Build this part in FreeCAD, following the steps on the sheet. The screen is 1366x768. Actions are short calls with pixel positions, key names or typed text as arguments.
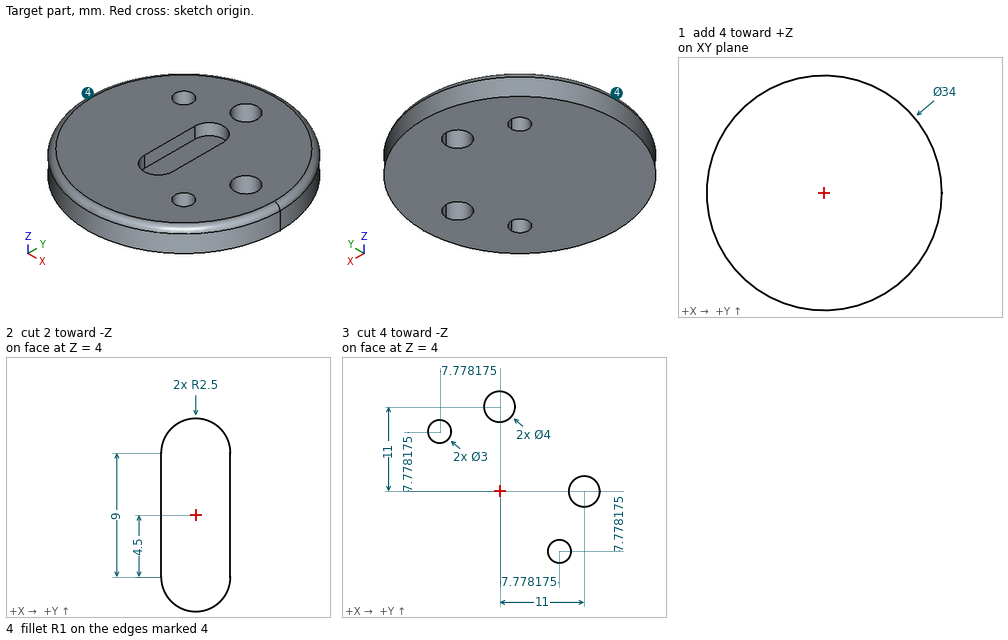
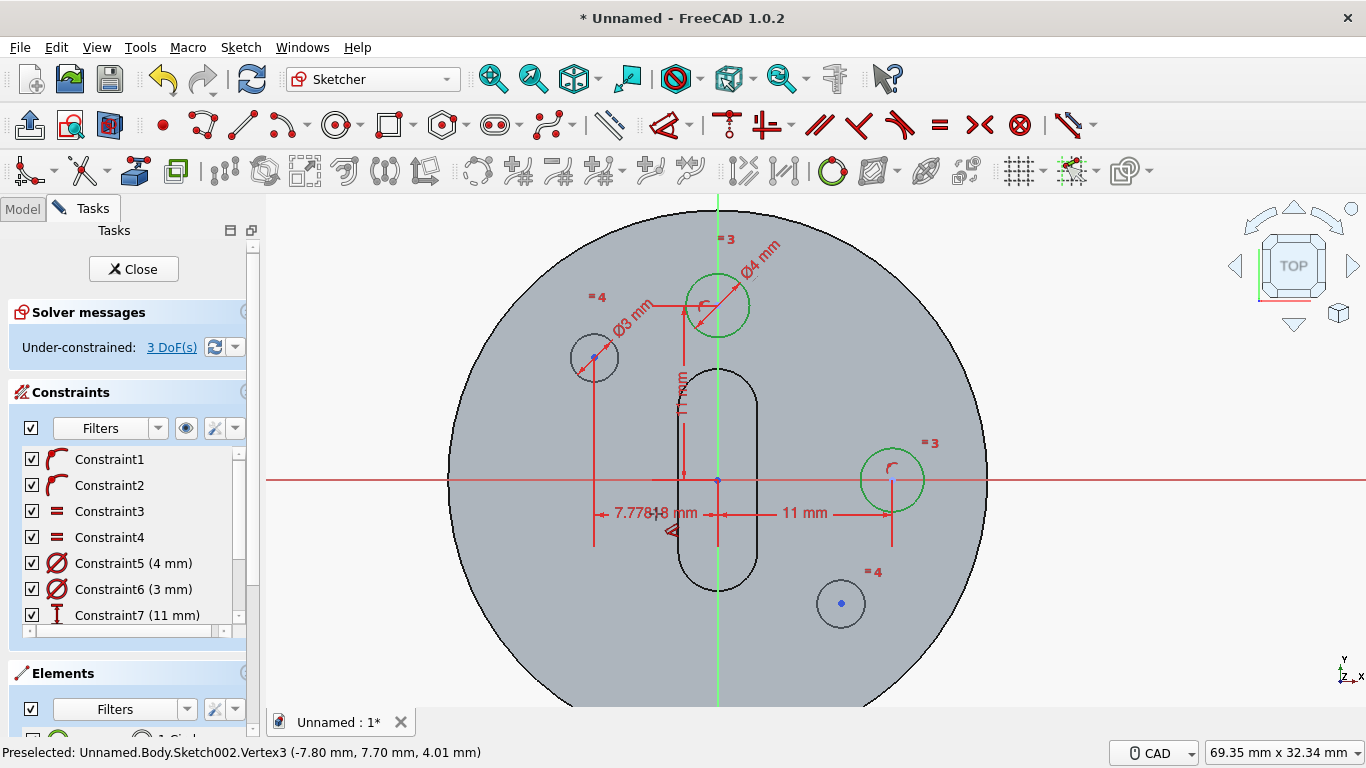
click(594, 358)
click(560, 419)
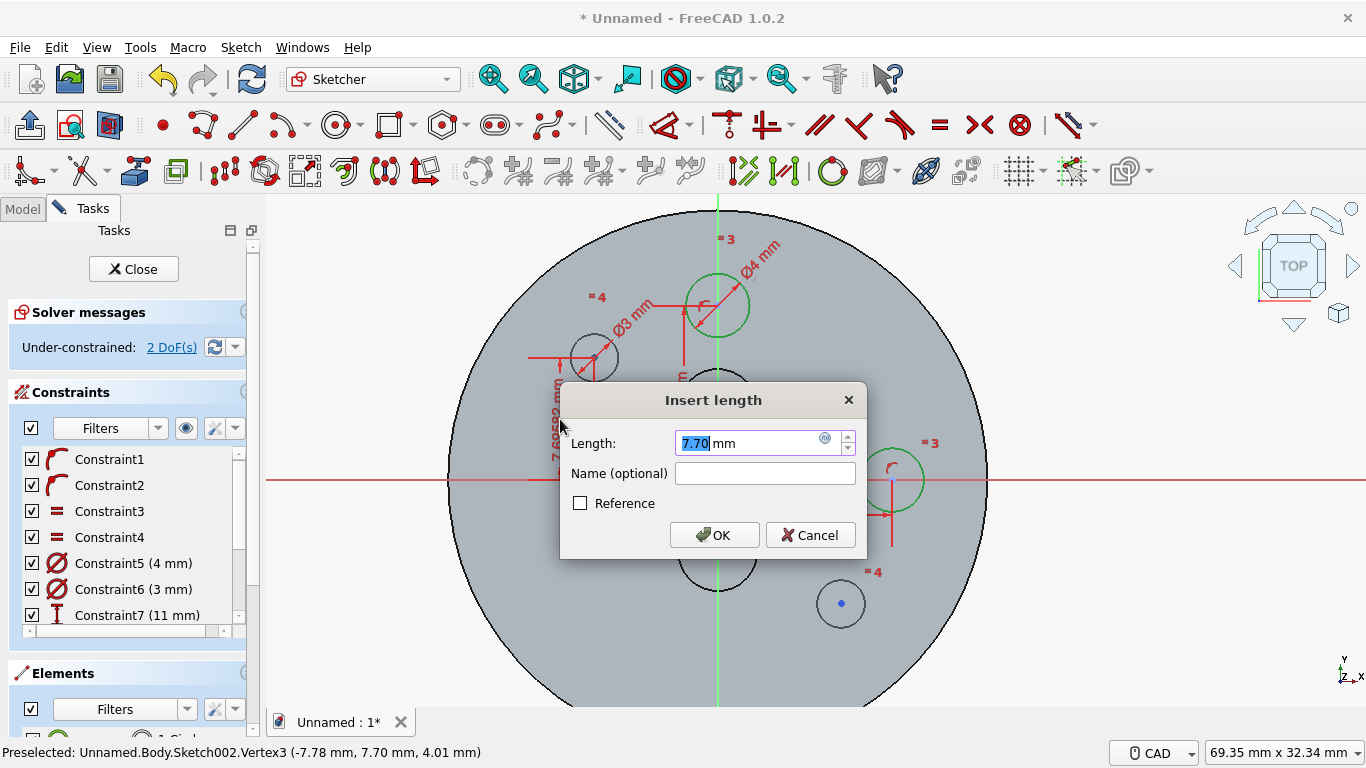
text(7.778175)
key(Return)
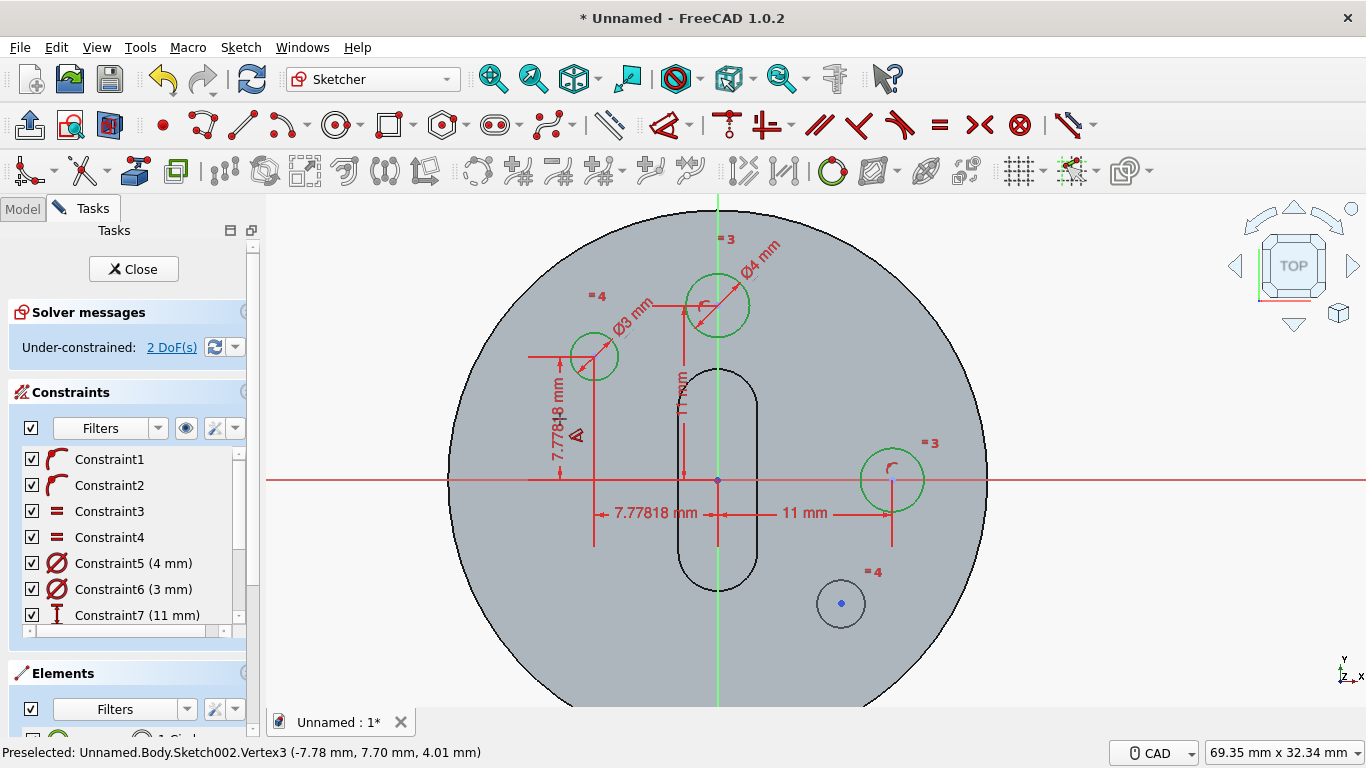
click(841, 604)
click(779, 638)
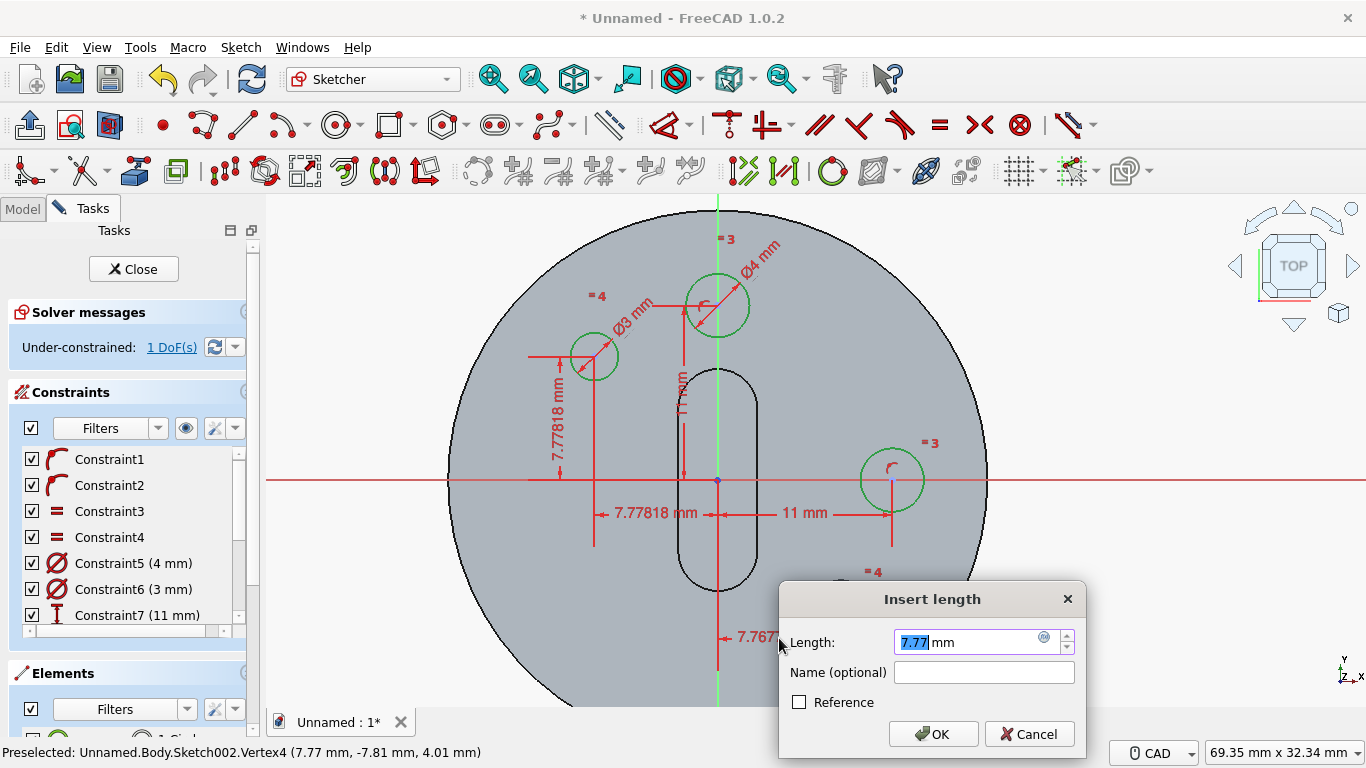
text(7.778175)
key(Return)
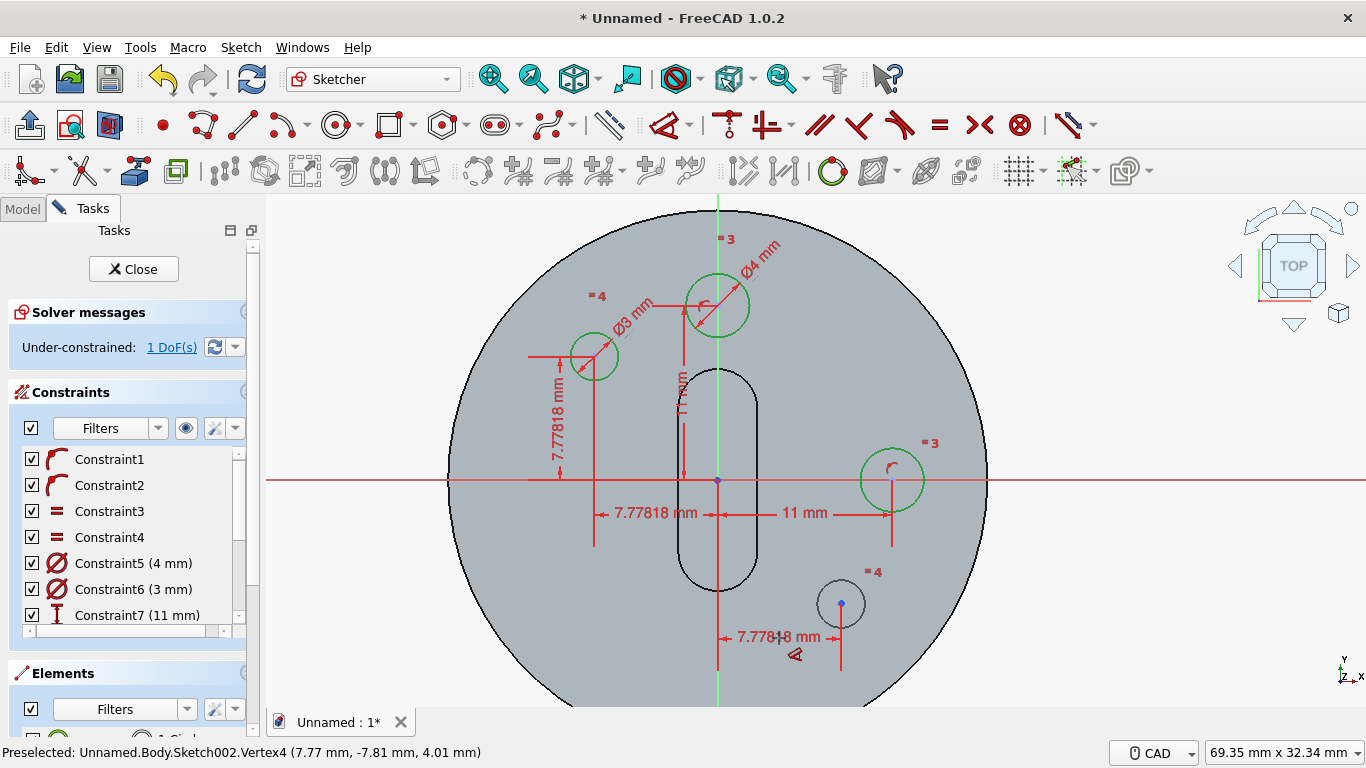
click(841, 604)
click(875, 542)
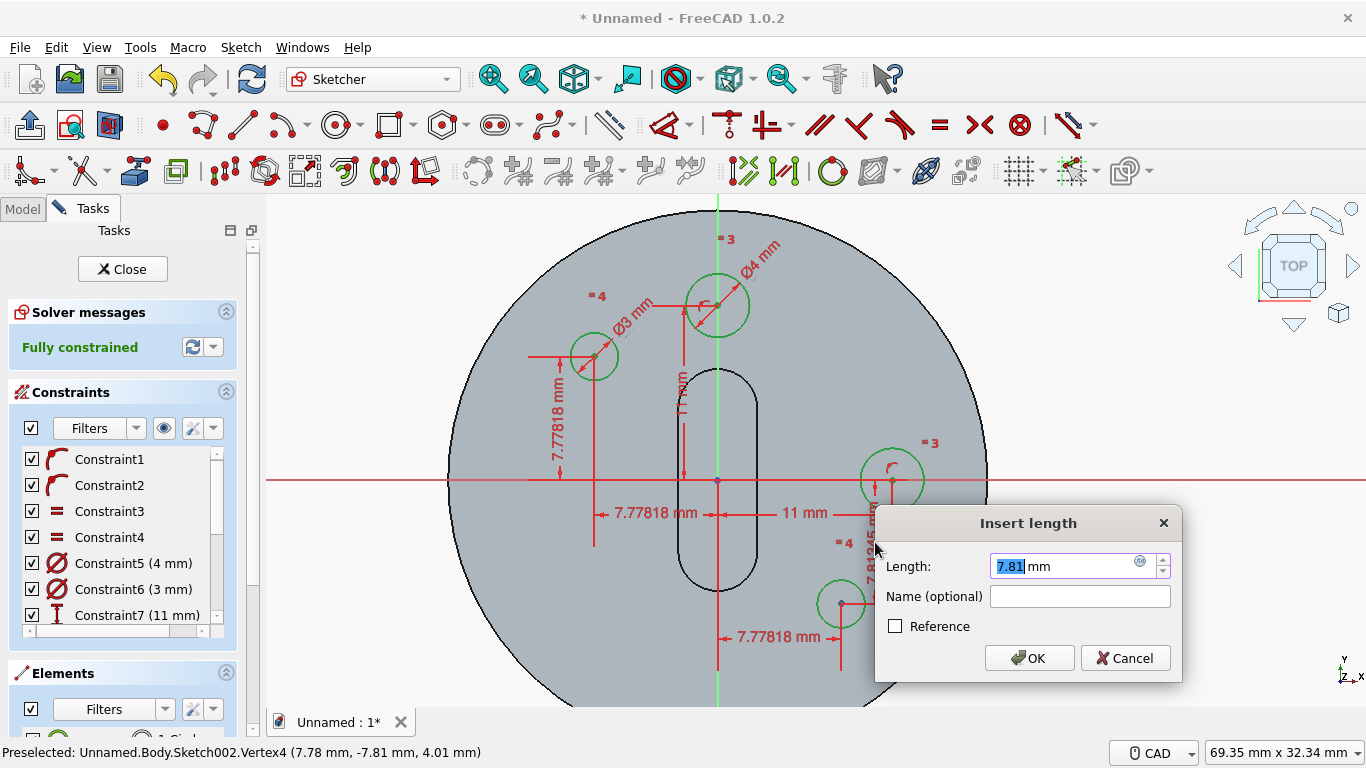
text(7.778175)
key(Return)
key(Escape)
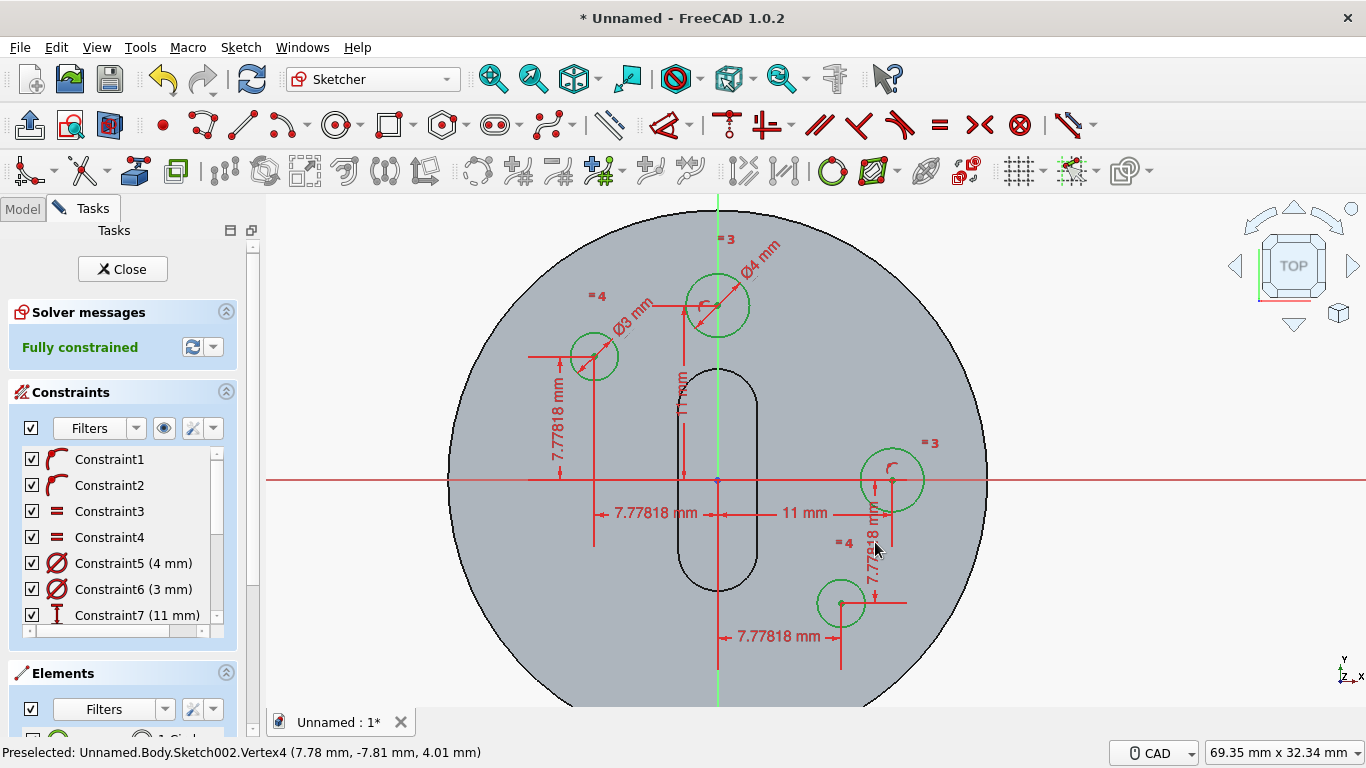
click(123, 269)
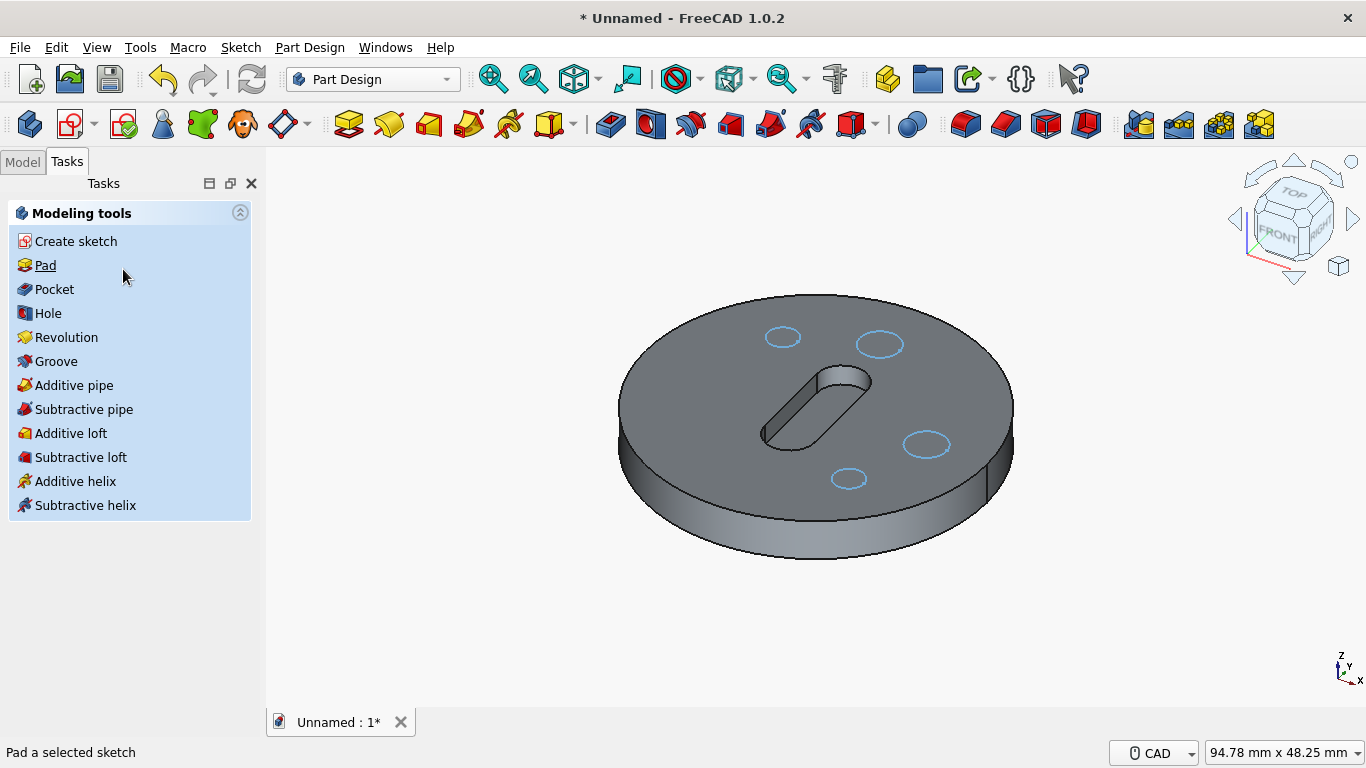
click(612, 124)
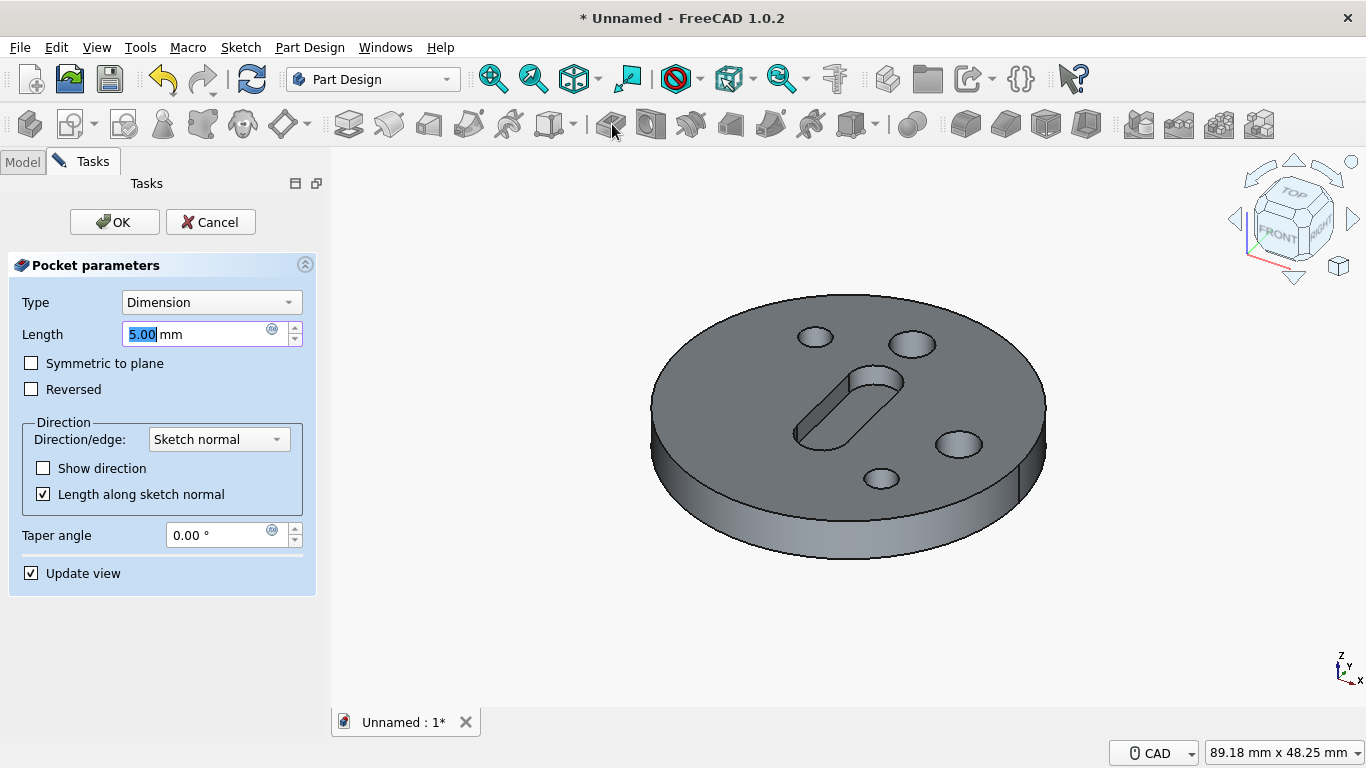
text(4)
key(Tab)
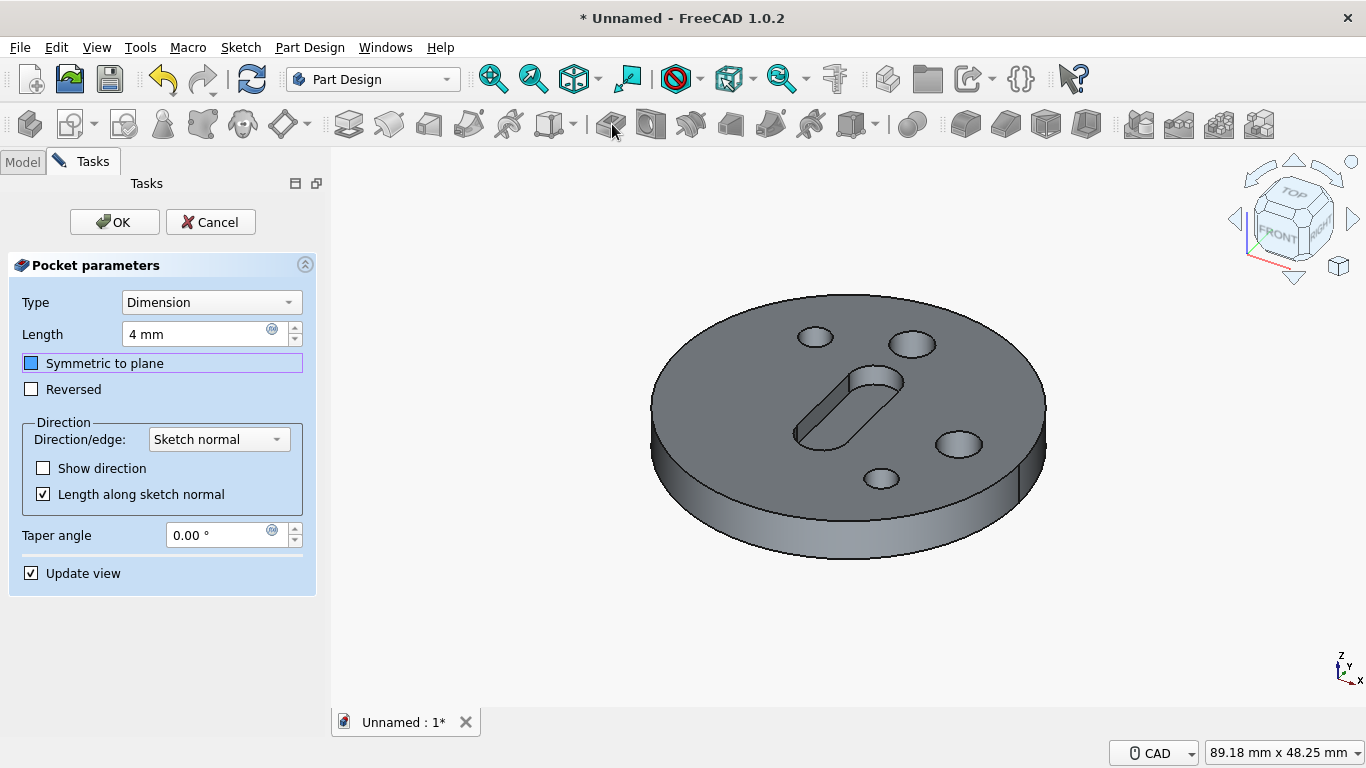
click(115, 222)